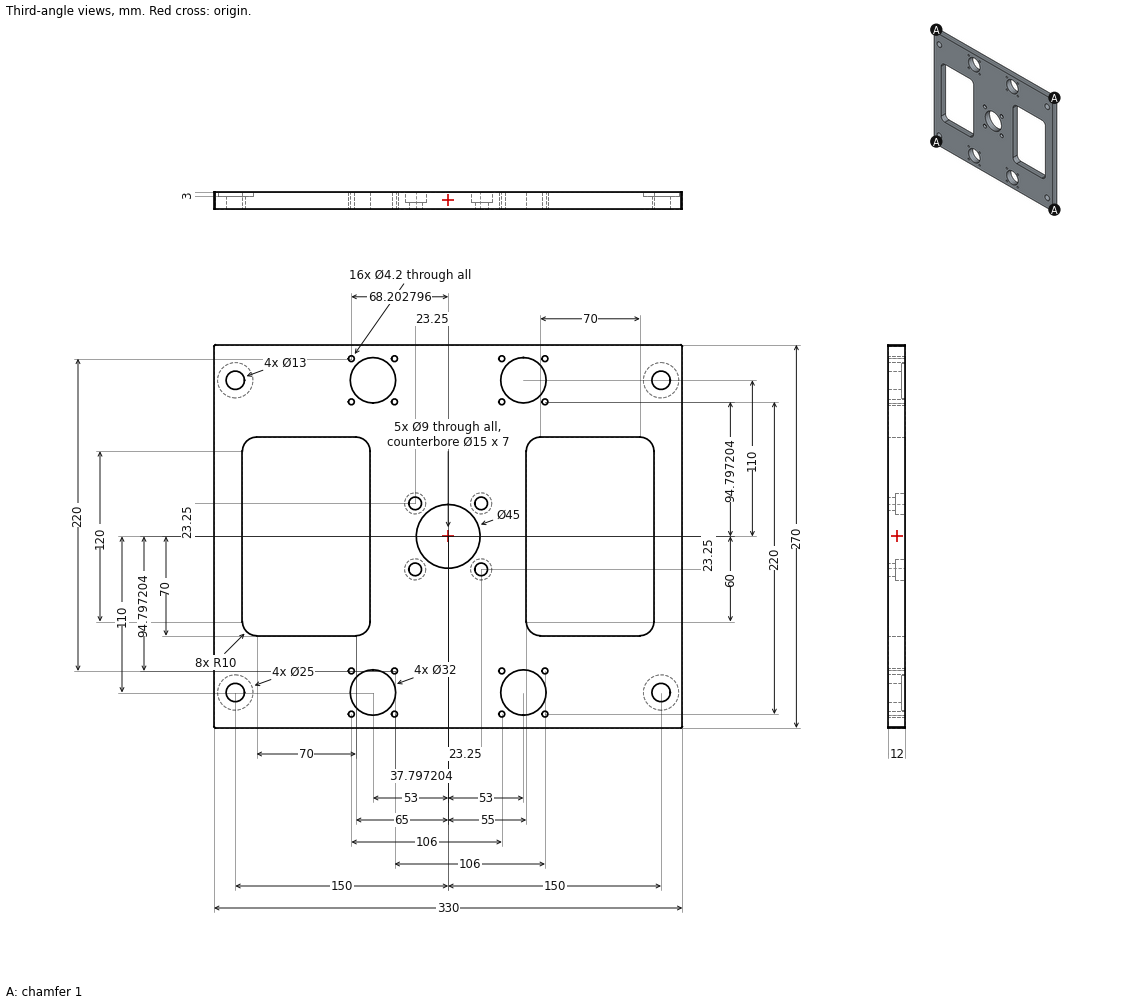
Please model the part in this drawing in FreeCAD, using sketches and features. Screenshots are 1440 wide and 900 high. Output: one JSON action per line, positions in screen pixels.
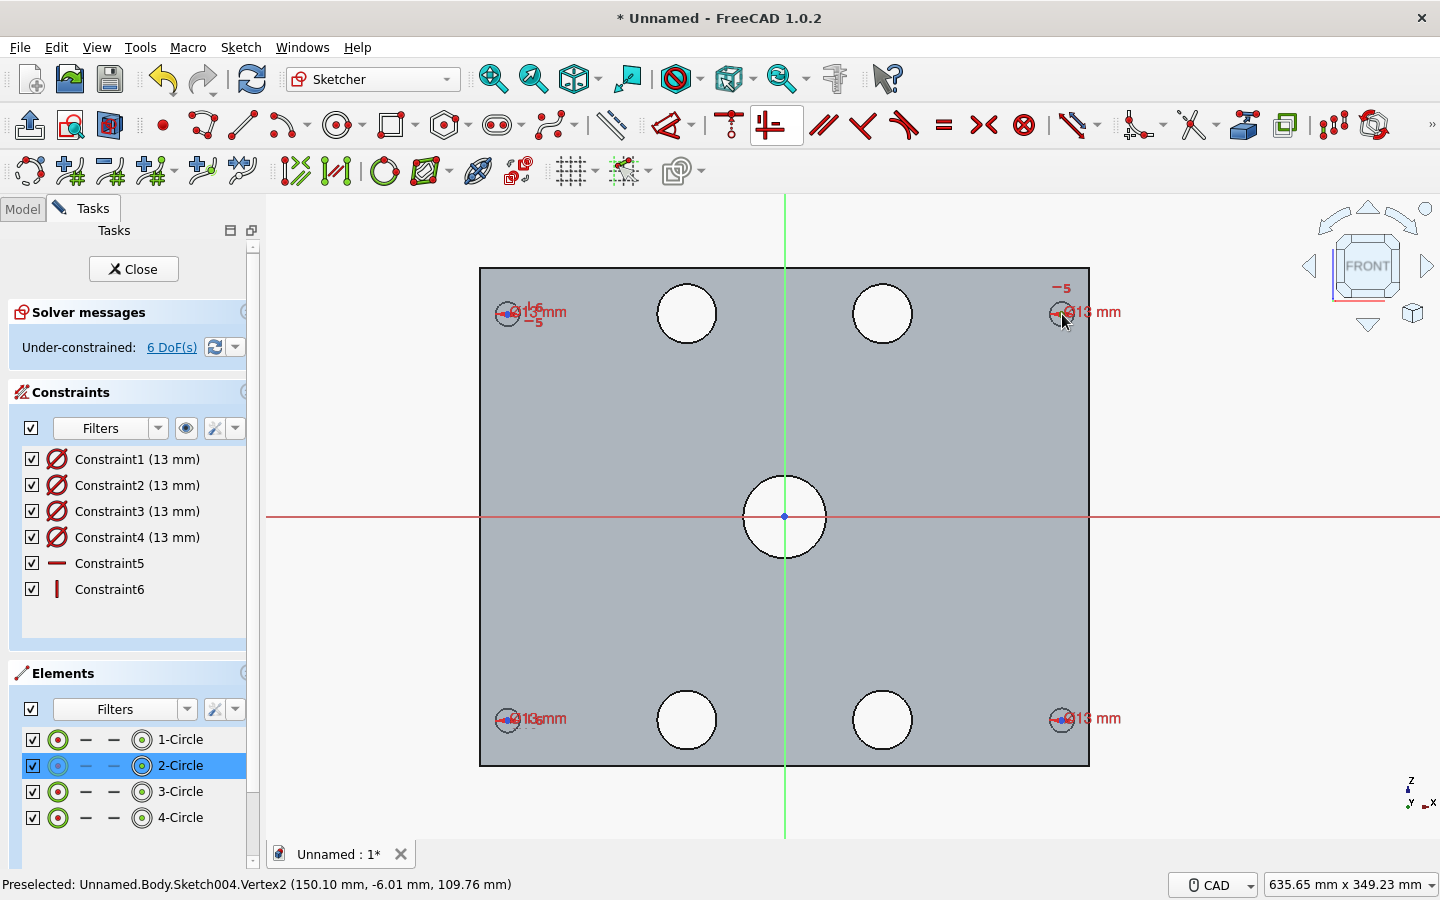
{"action": "left_click", "coordinate": [1062, 720]}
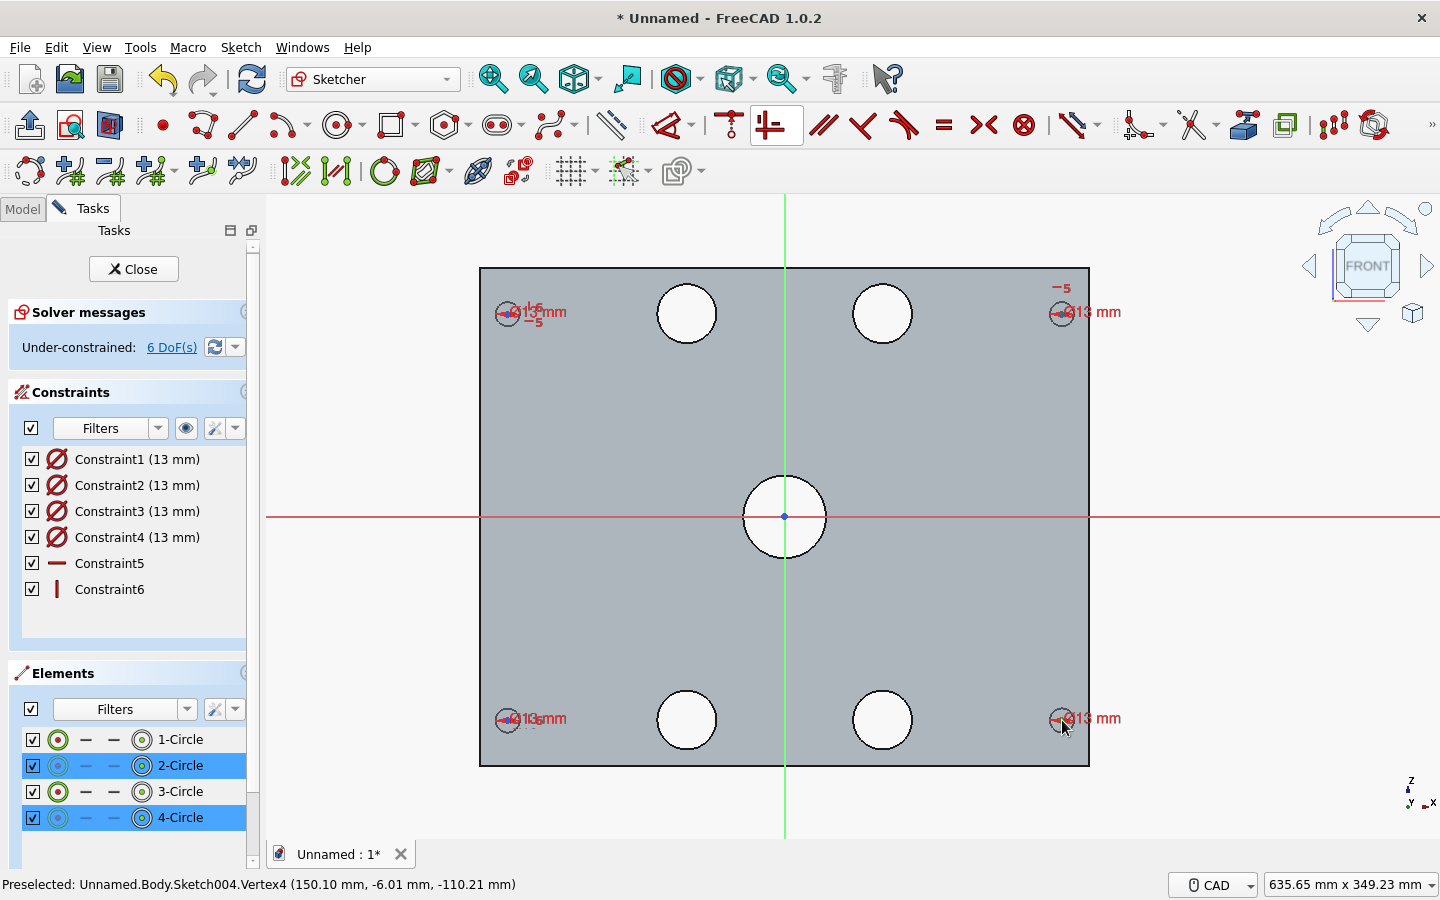
{"action": "left_click", "coordinate": [798, 126]}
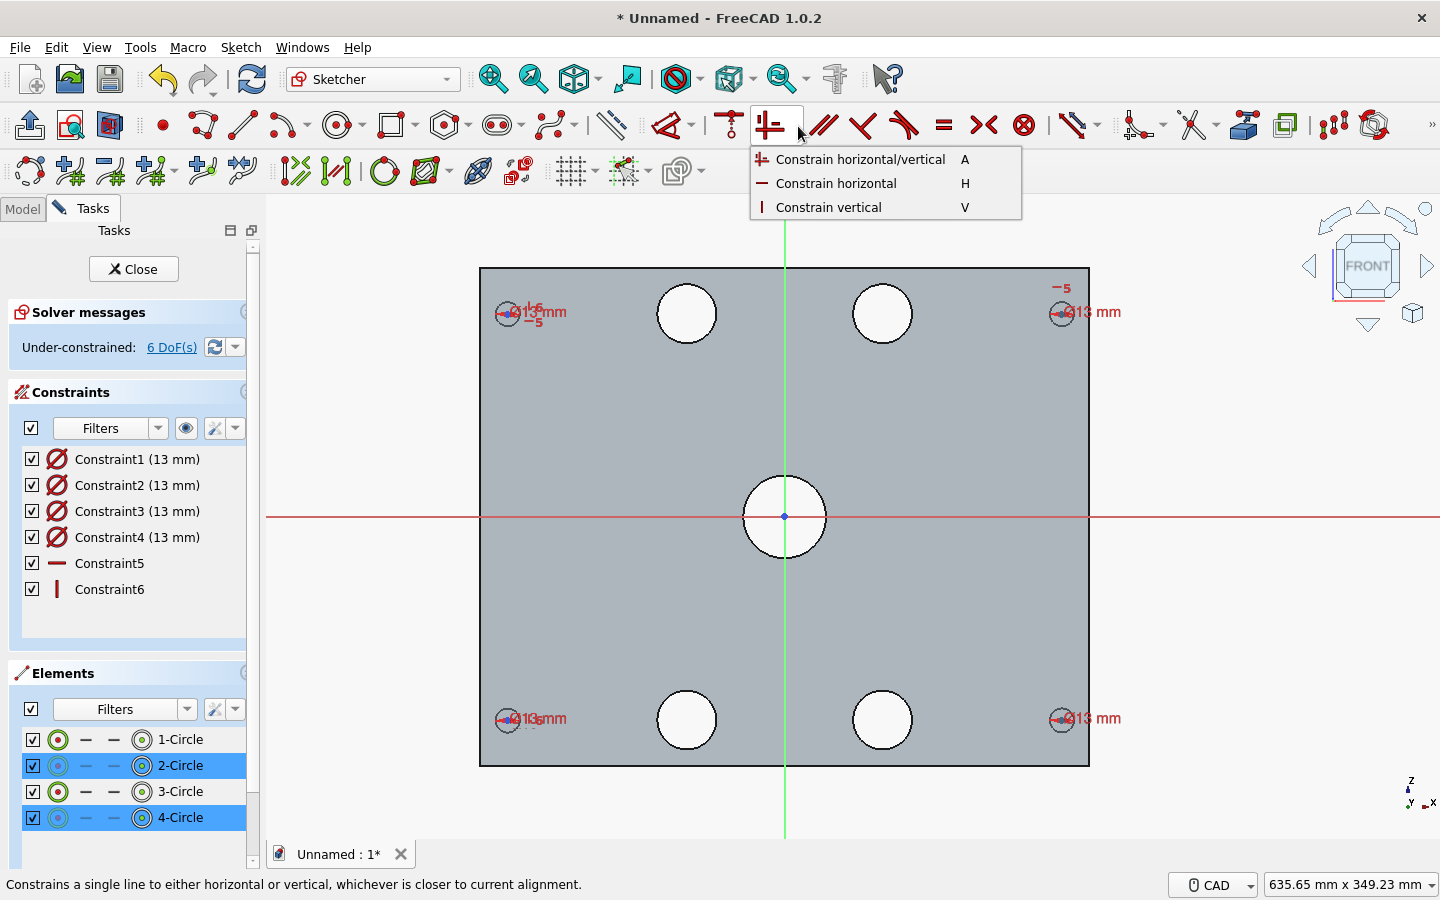
{"action": "left_click", "coordinate": [886, 207]}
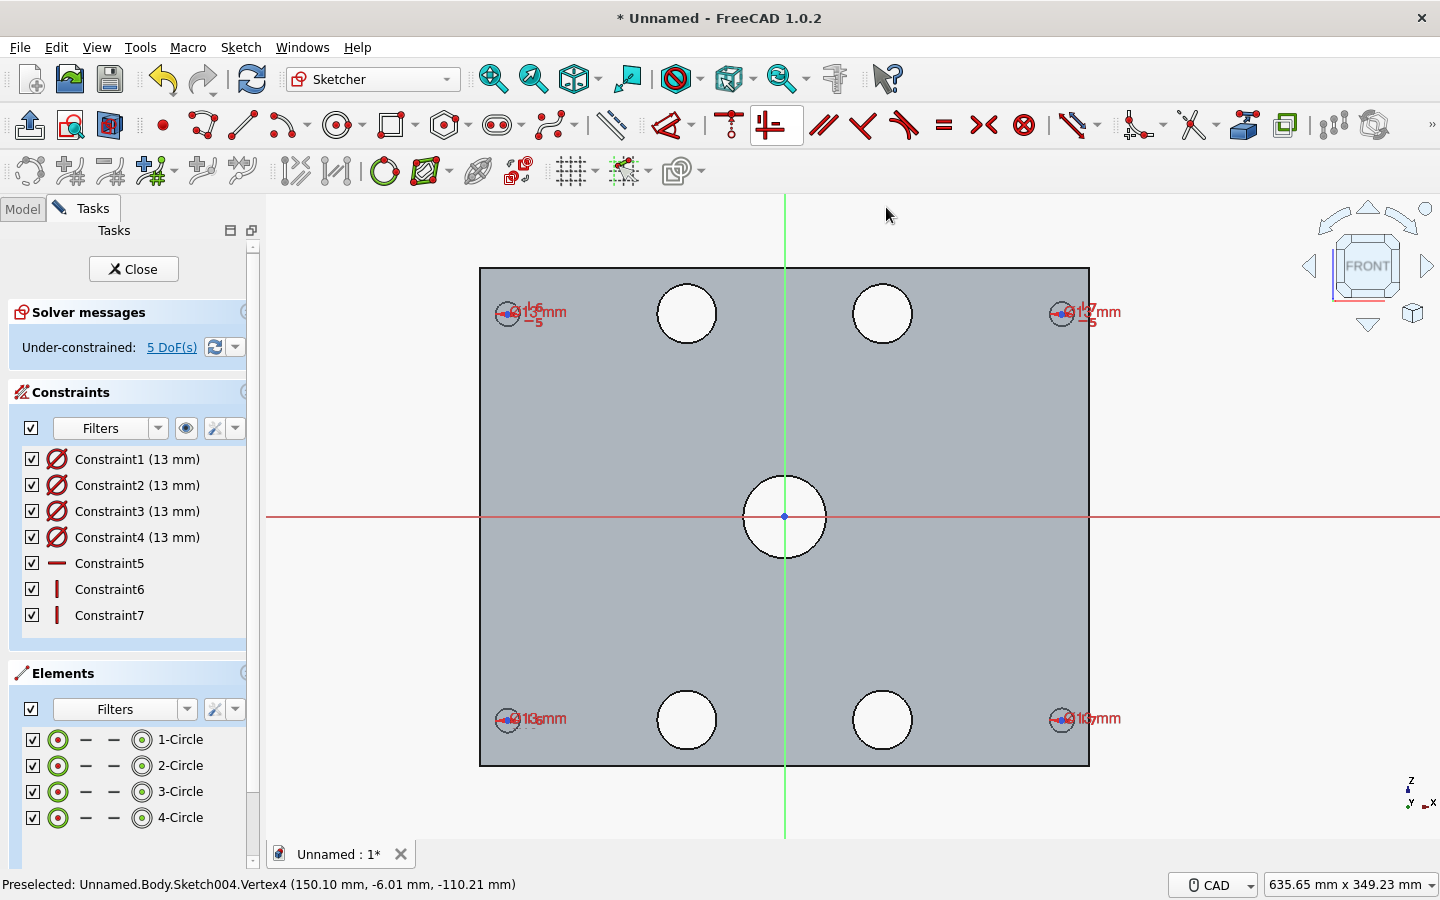
{"action": "left_click", "coordinate": [508, 721]}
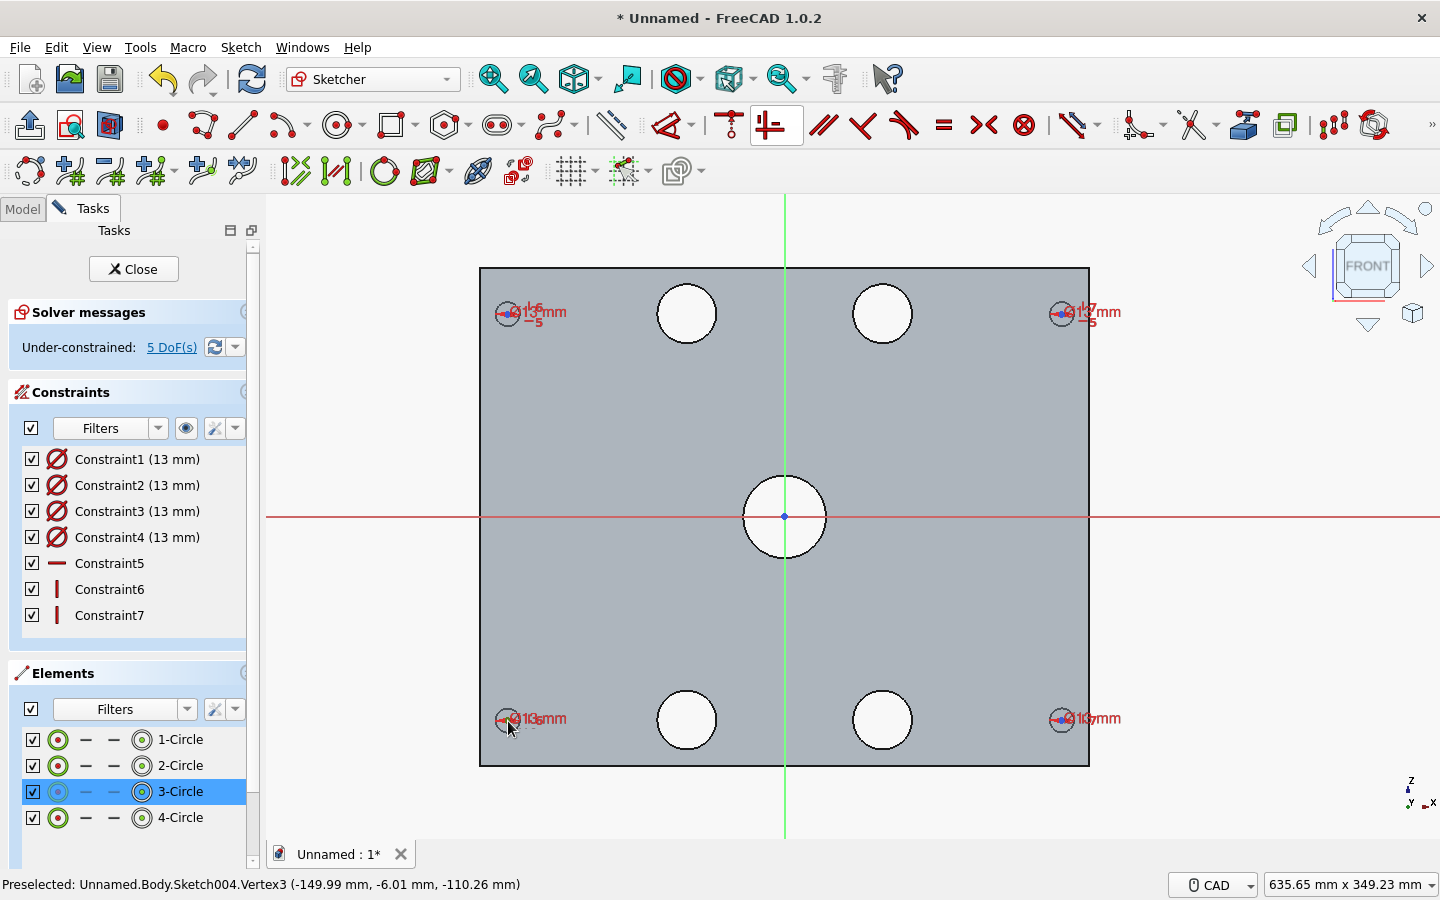
{"action": "left_click", "coordinate": [1062, 720]}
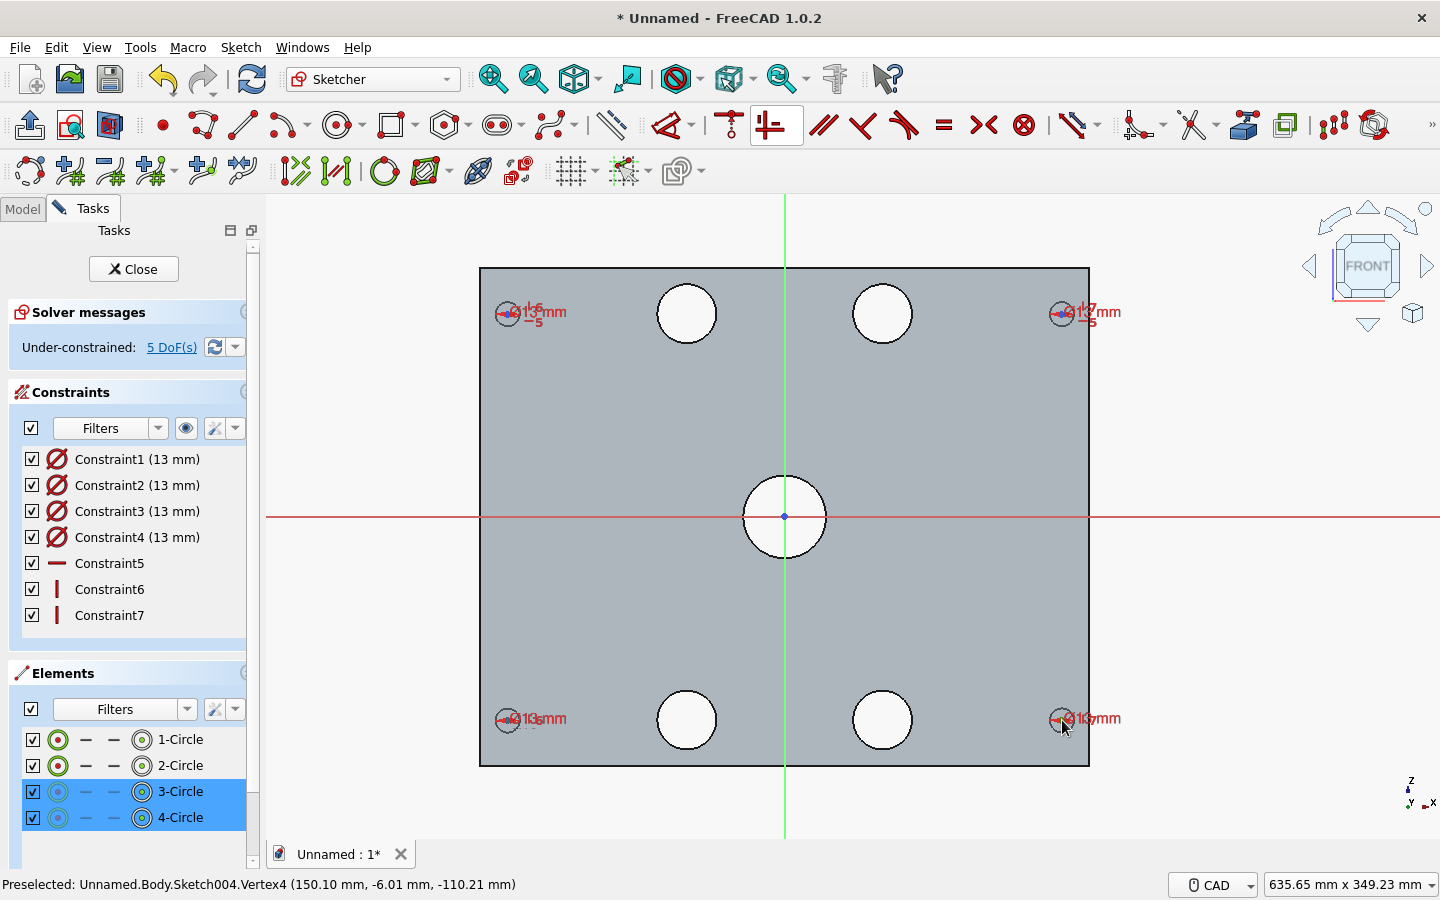
{"action": "key", "text": "h"}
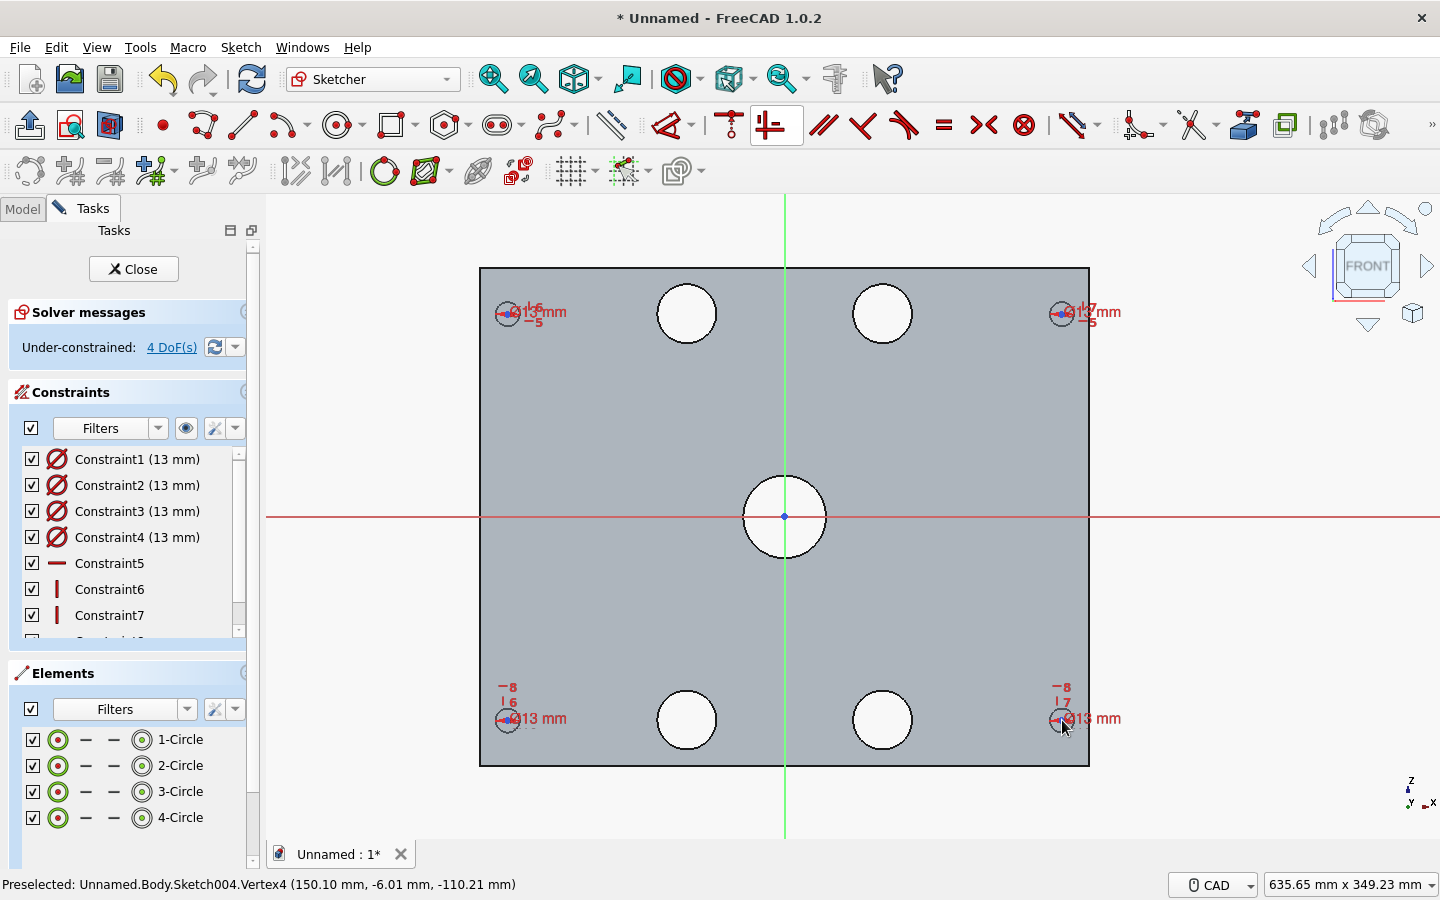
{"action": "key", "text": "d"}